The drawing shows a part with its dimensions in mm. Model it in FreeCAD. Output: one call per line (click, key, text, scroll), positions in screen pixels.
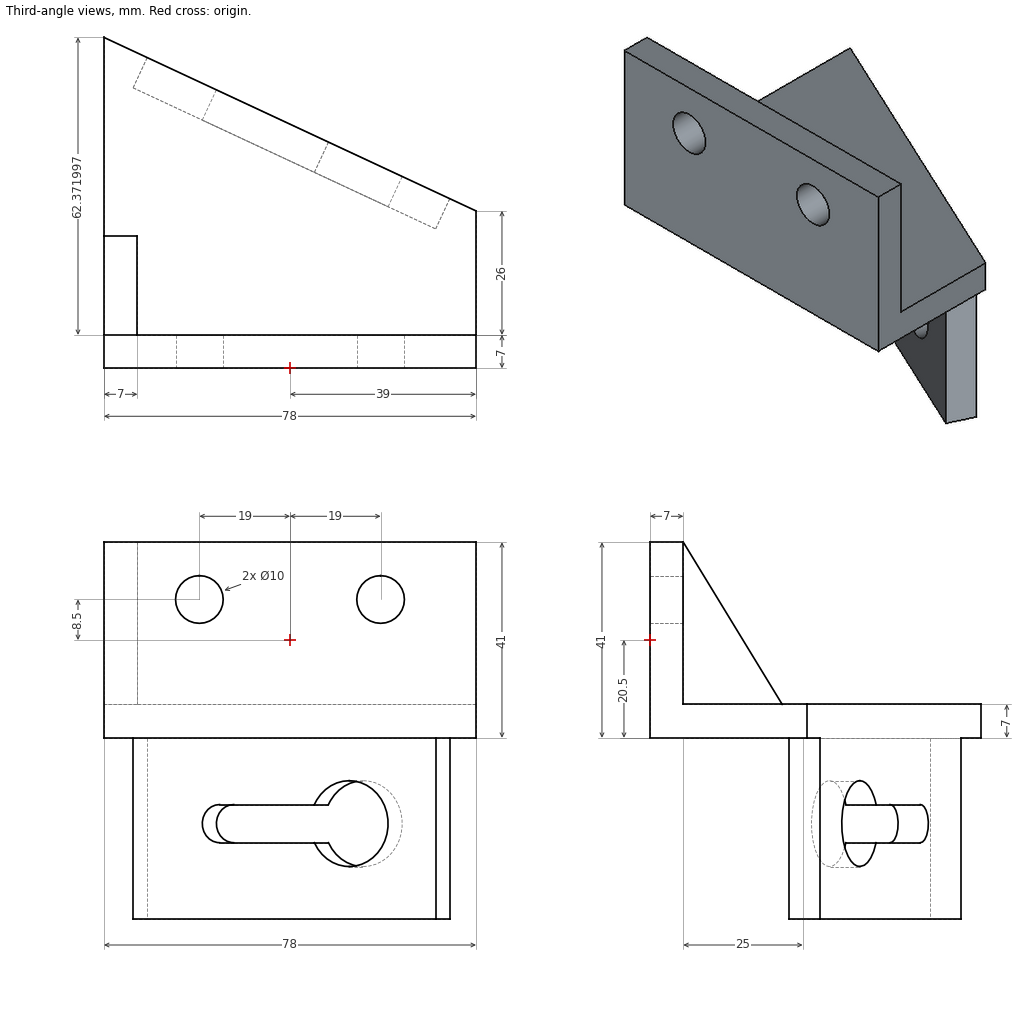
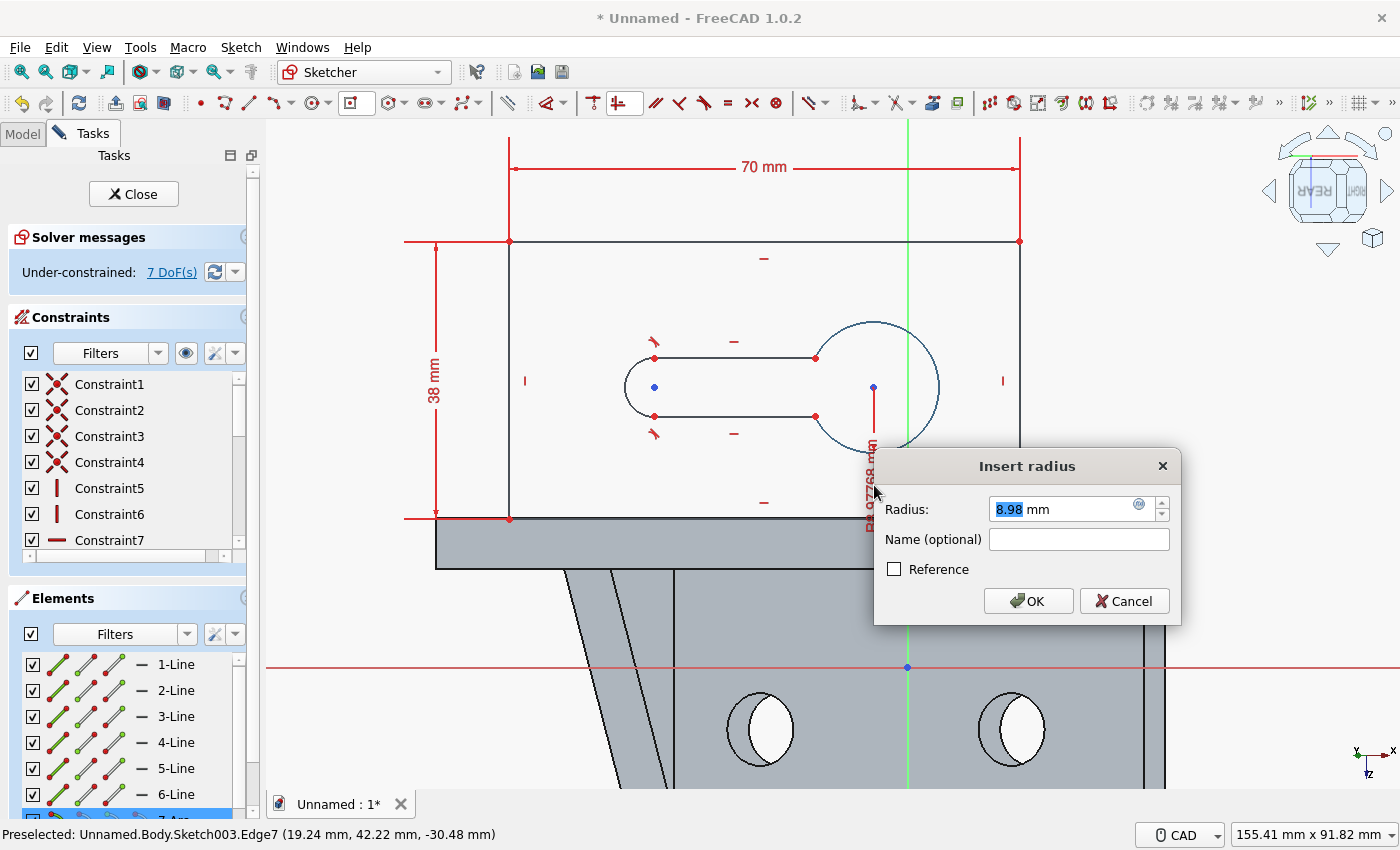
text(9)
key(Return)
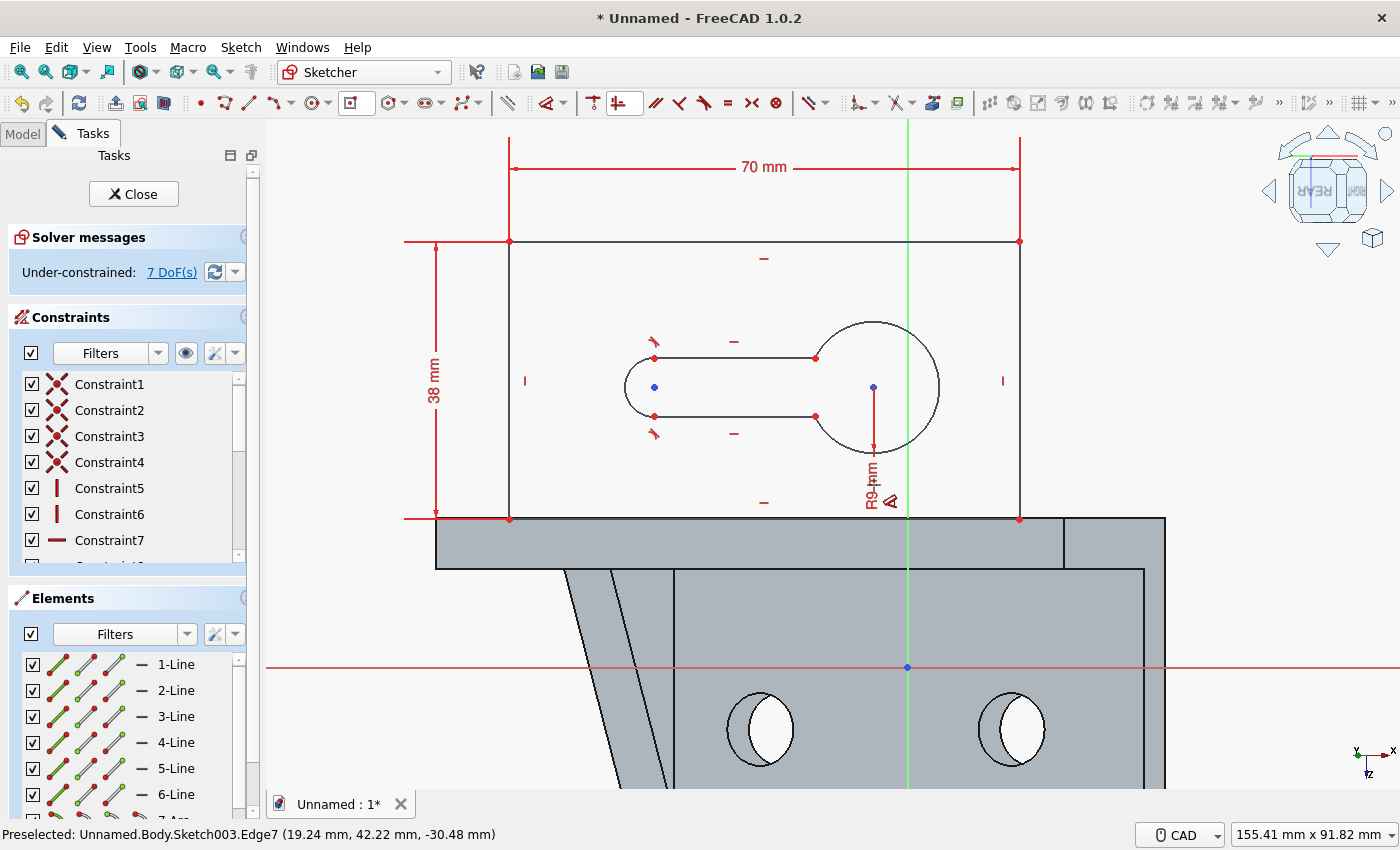
scroll(631, 370, up, 2)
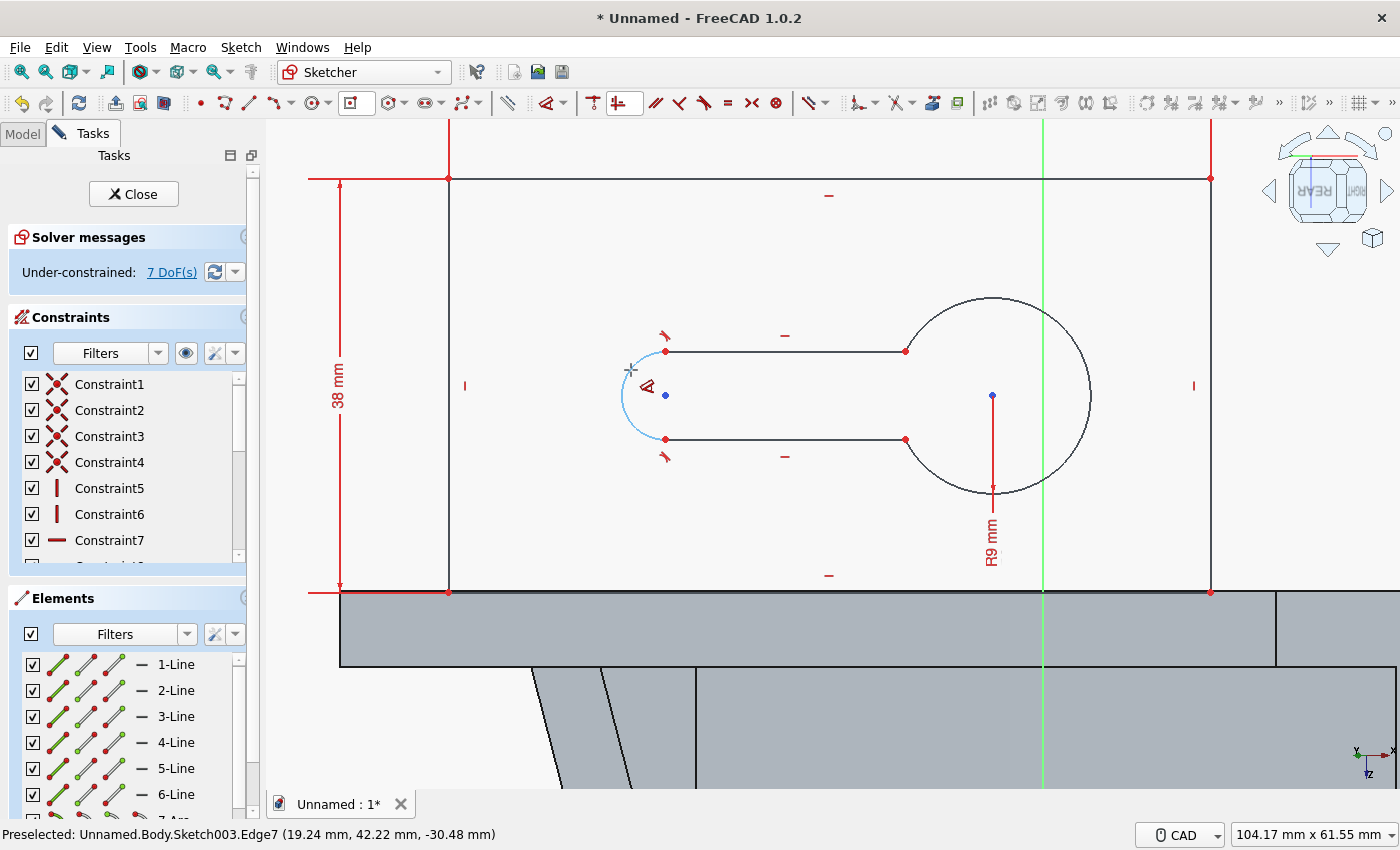
click(630, 370)
click(604, 351)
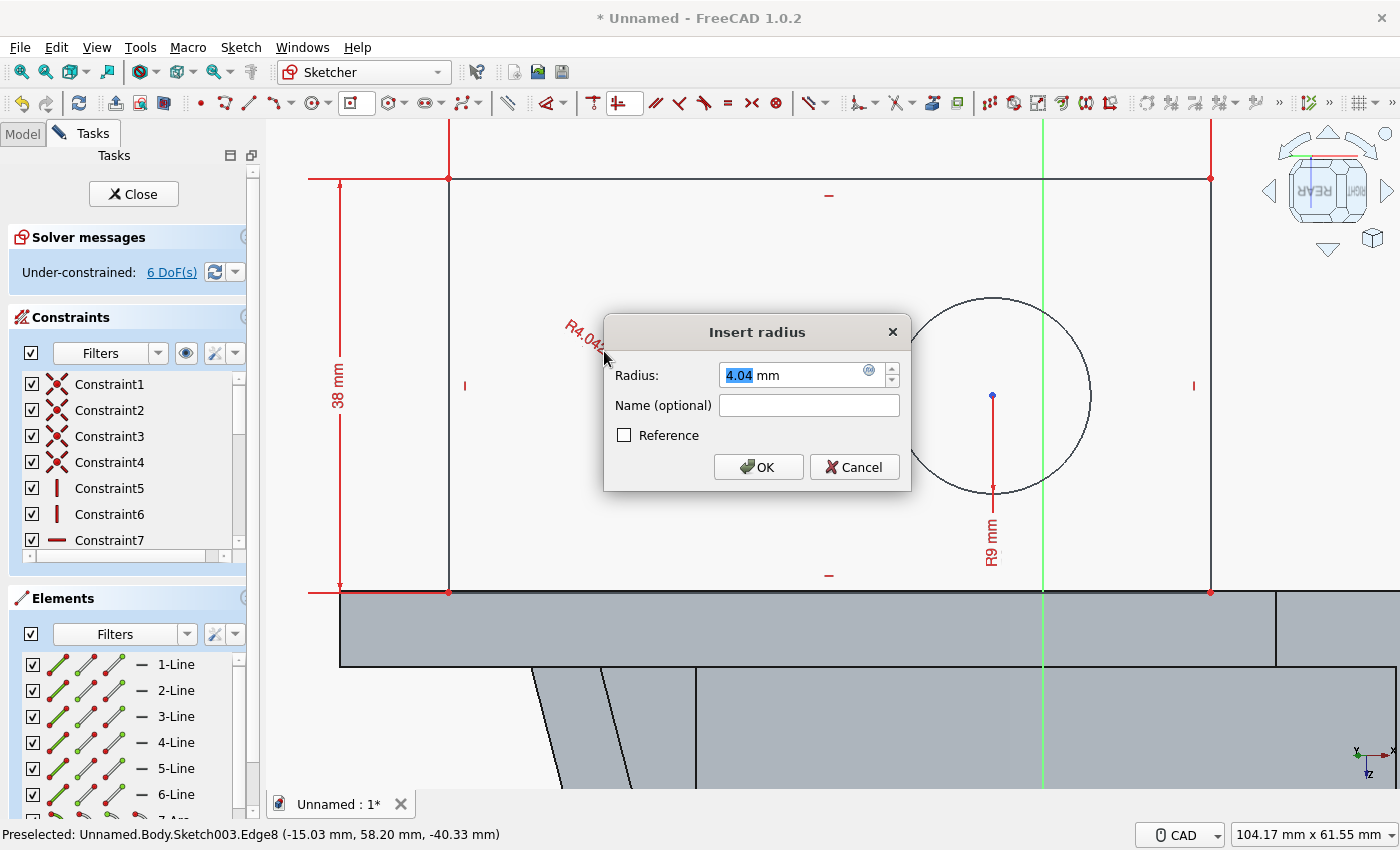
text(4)
key(Return)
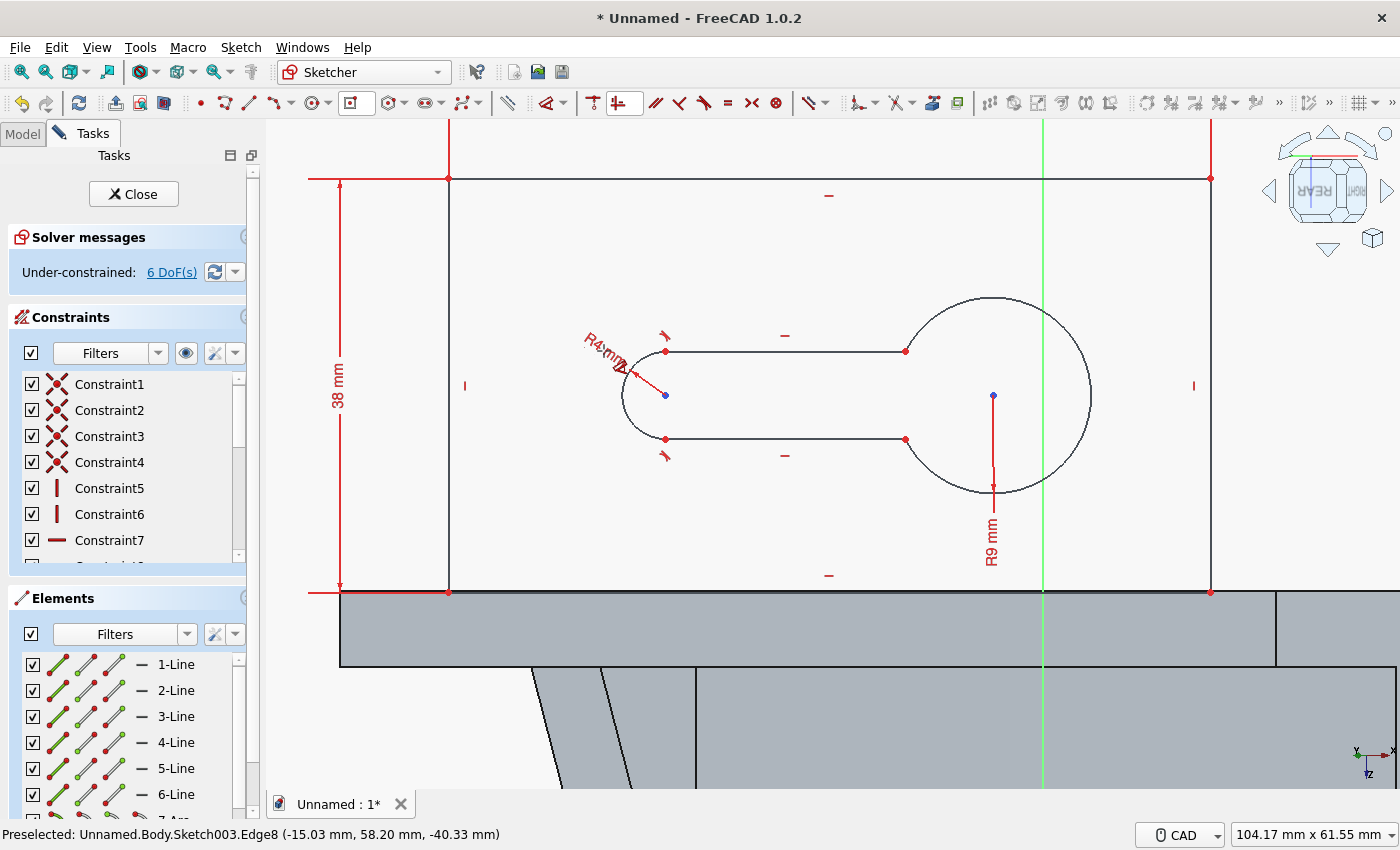
click(449, 179)
click(415, 470)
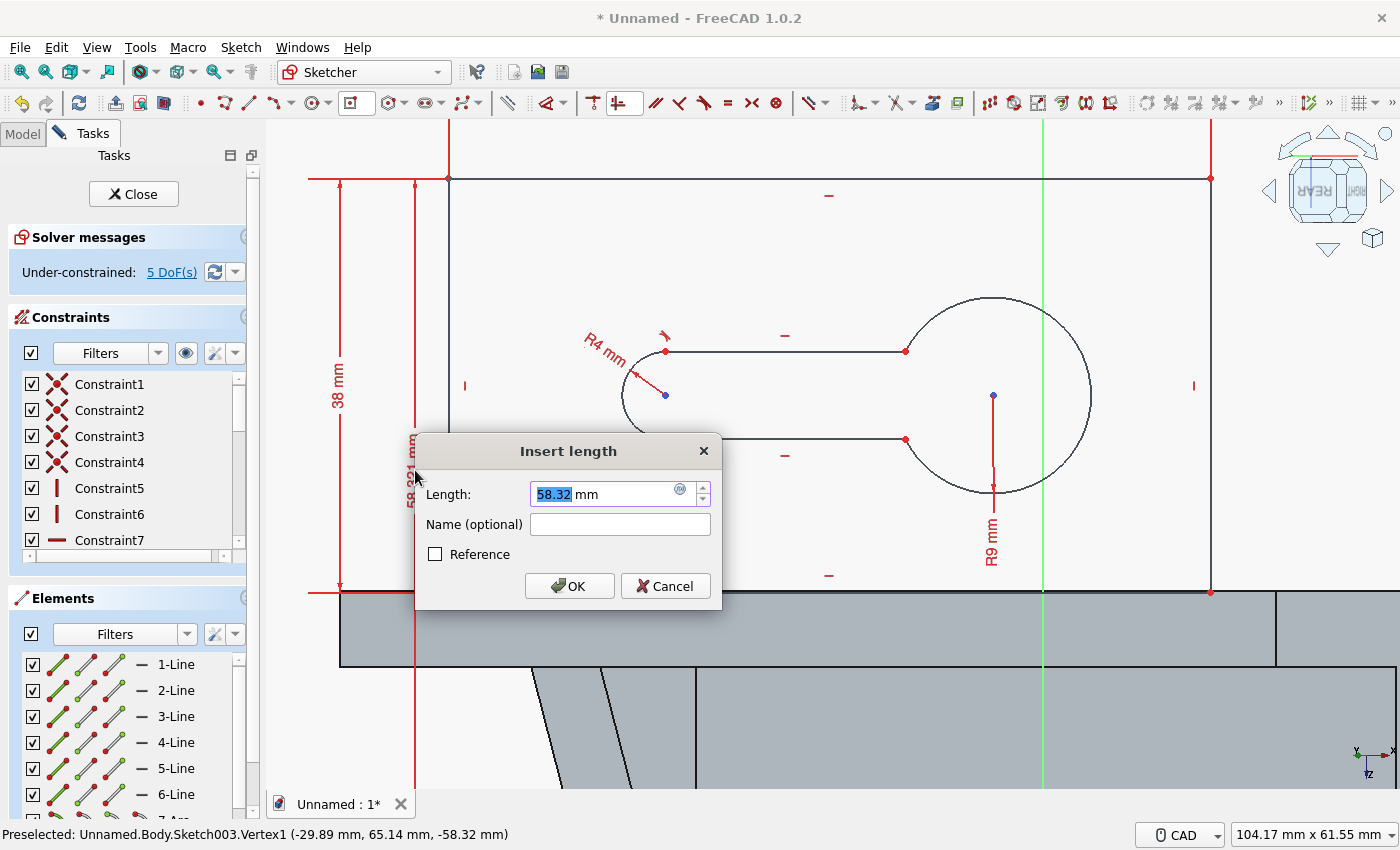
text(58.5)
key(Return)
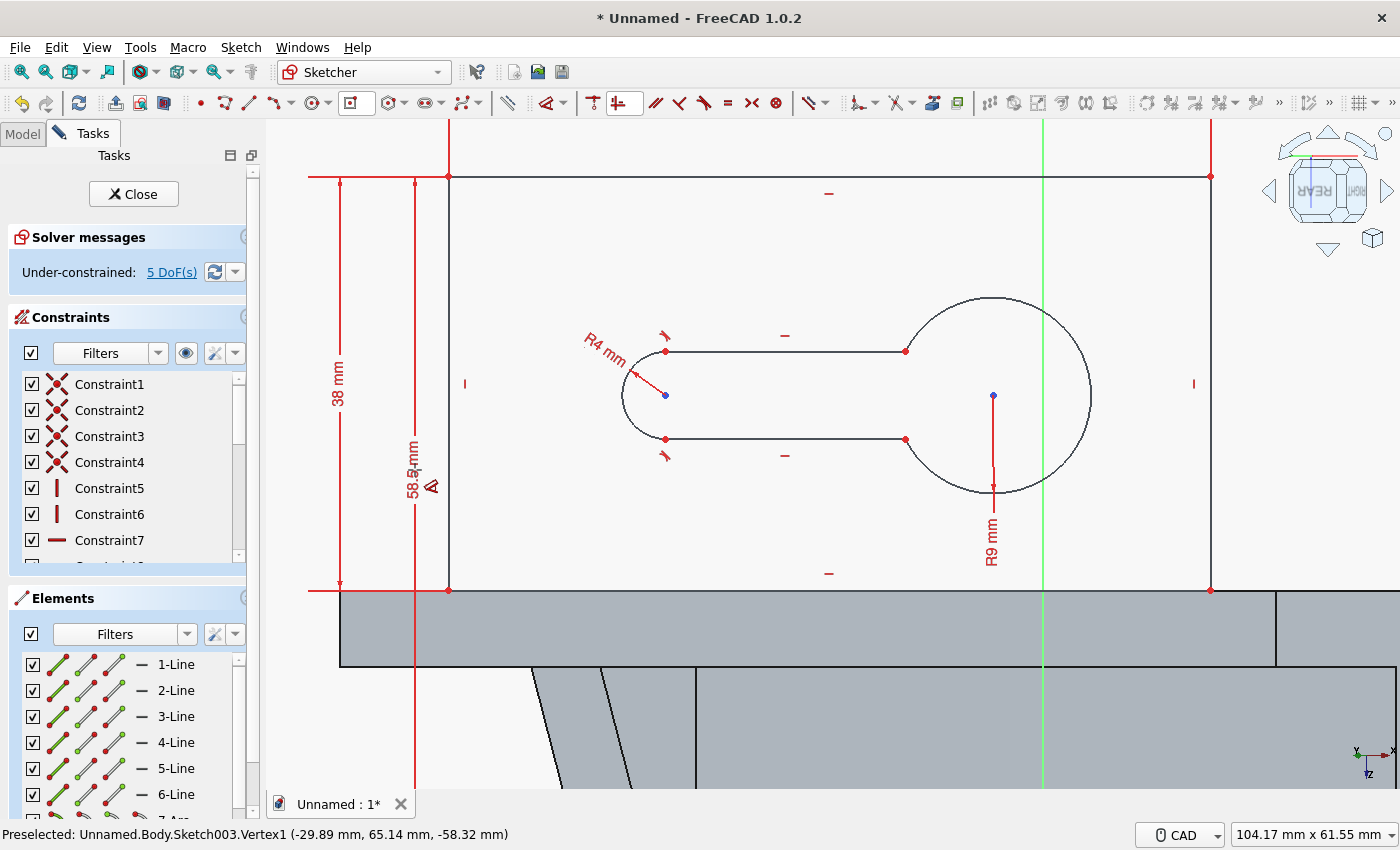
click(666, 352)
click(1077, 556)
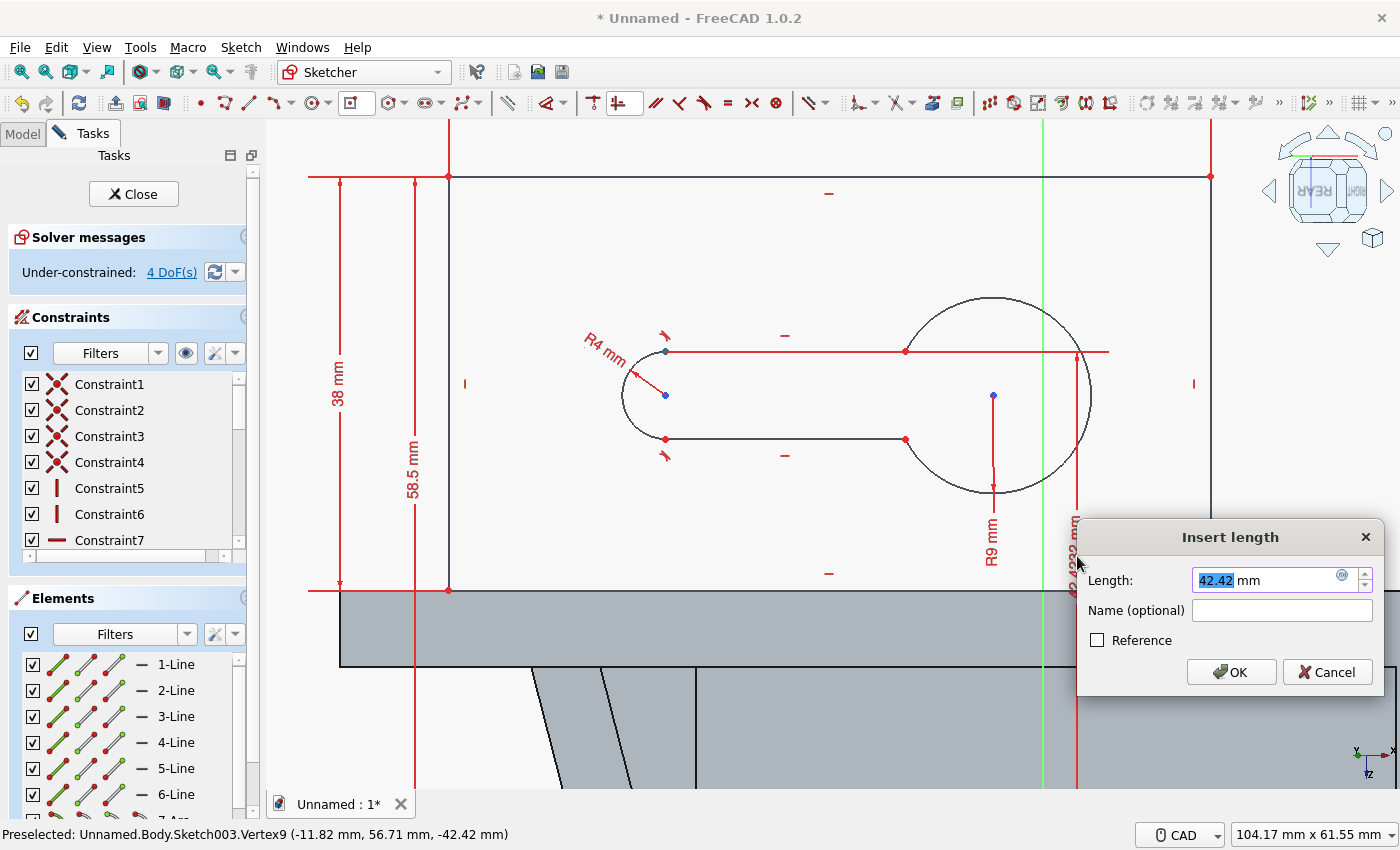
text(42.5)
key(Return)